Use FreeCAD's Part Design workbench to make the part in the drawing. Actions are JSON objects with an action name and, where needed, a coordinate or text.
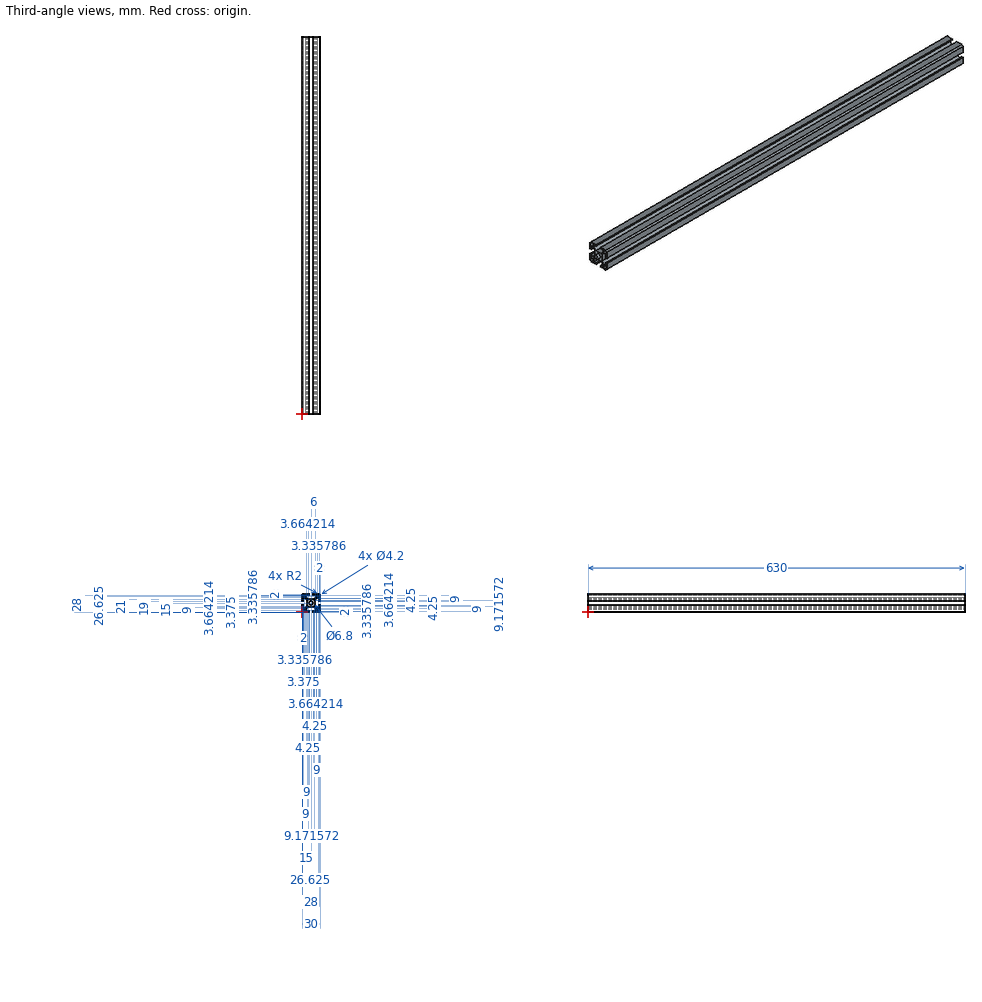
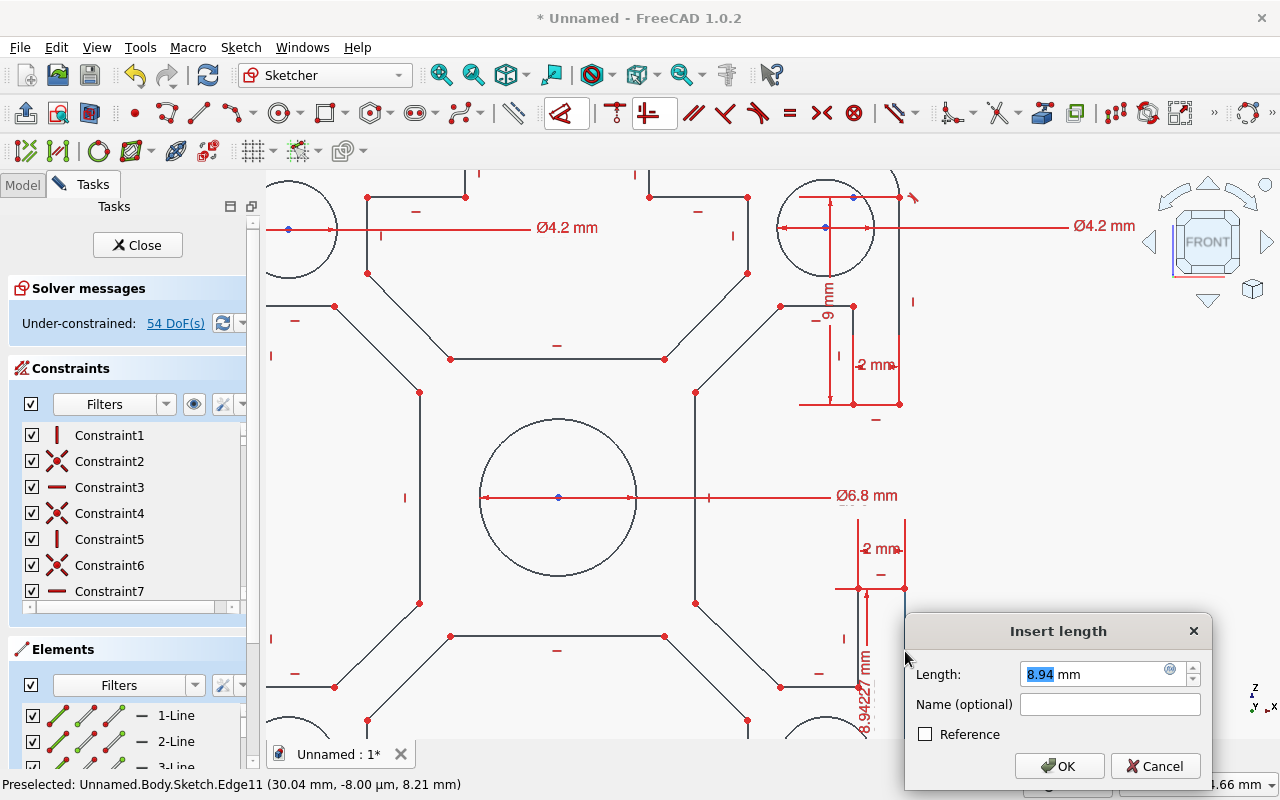
{"action": "type", "text": "9"}
{"action": "key", "text": "Return"}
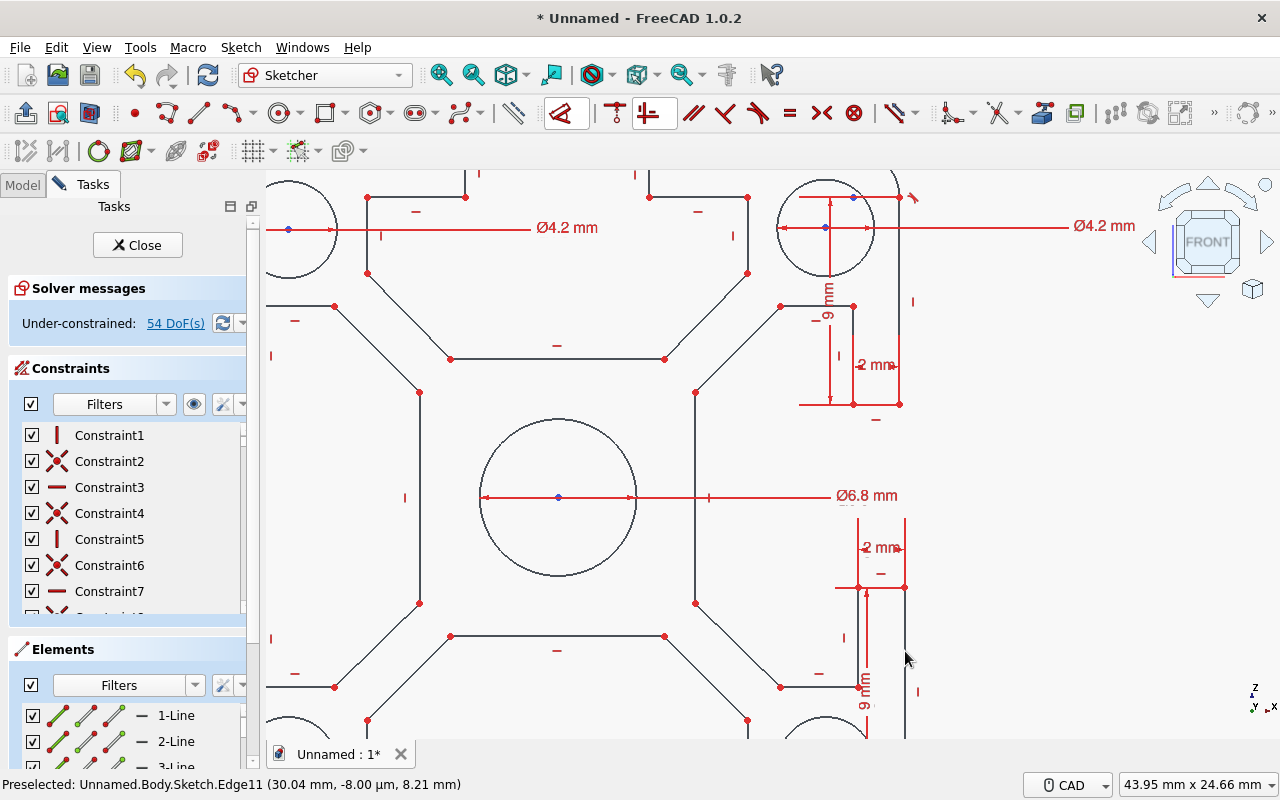
{"action": "scroll", "coordinate": [883, 405], "scroll_direction": "down", "scroll_amount": 3}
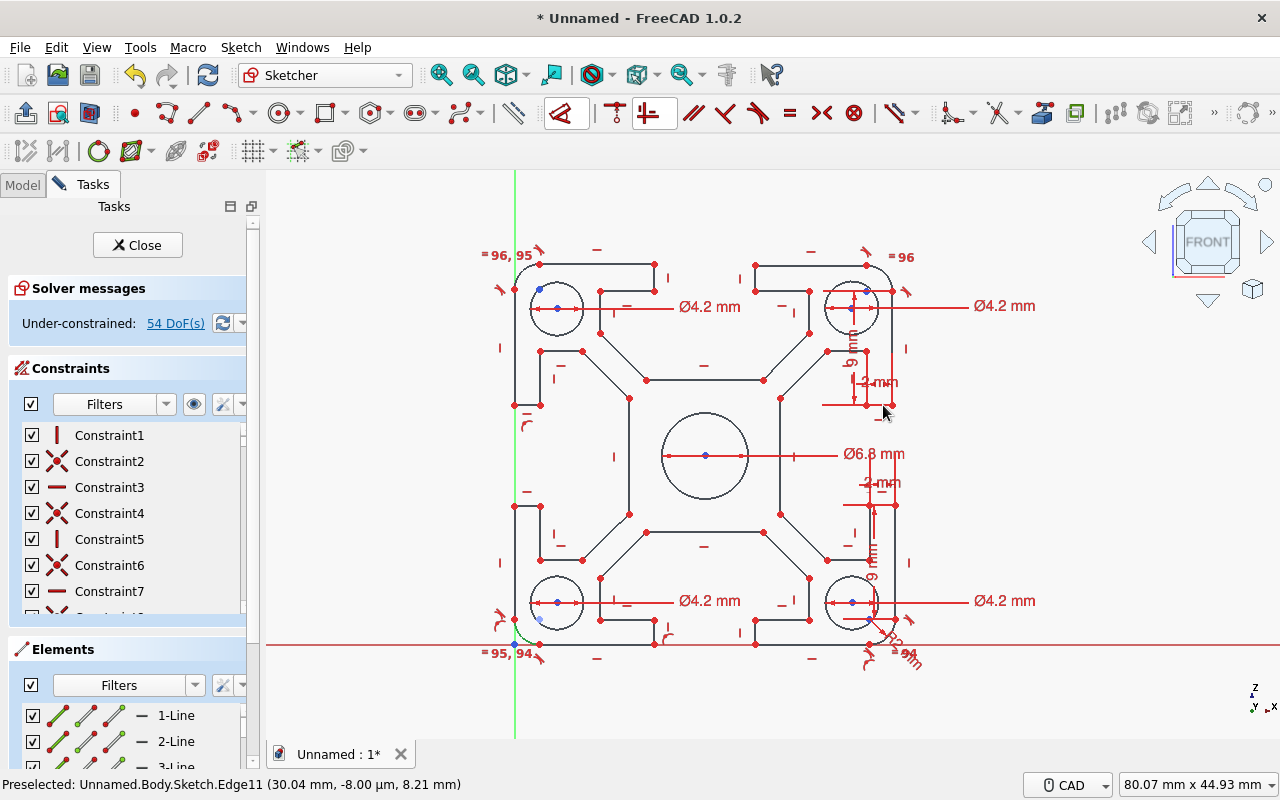
{"action": "left_click", "coordinate": [835, 645]}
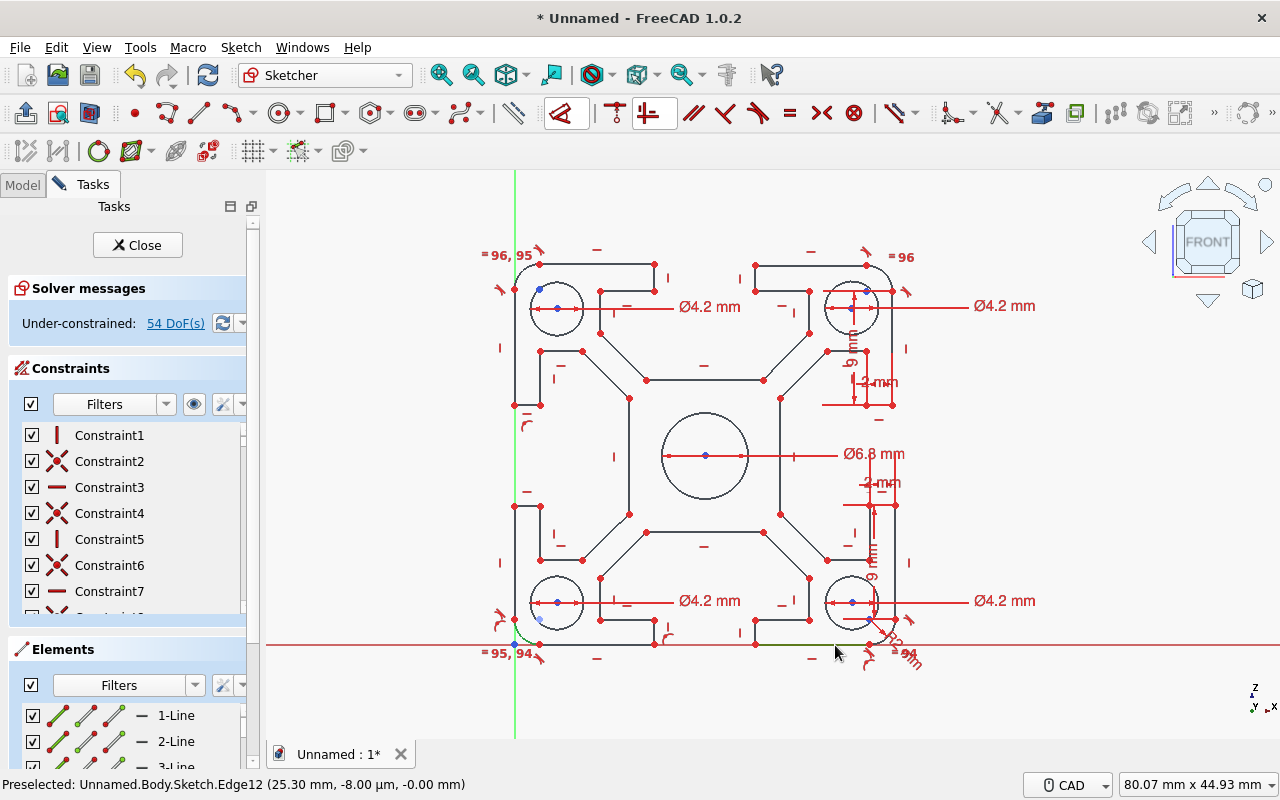
{"action": "key", "text": "l"}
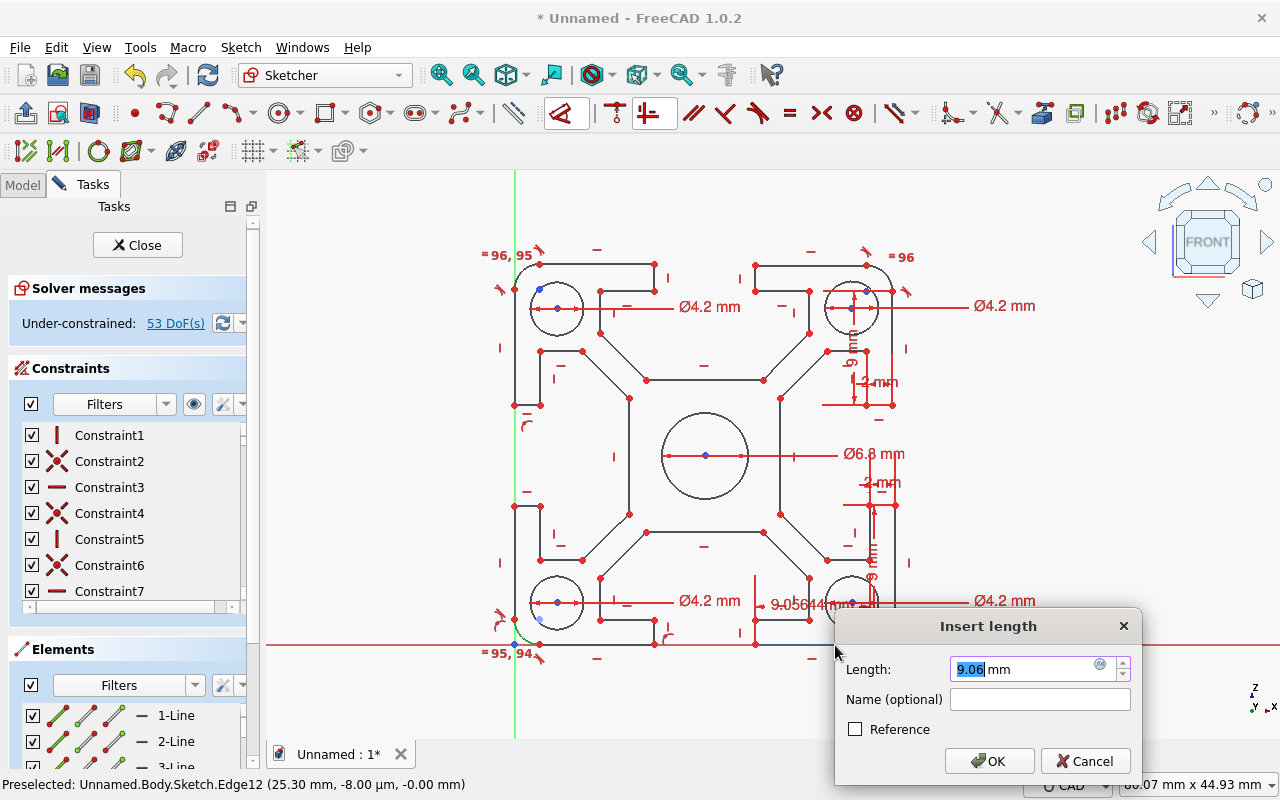
{"action": "type", "text": "9"}
{"action": "key", "text": "Return"}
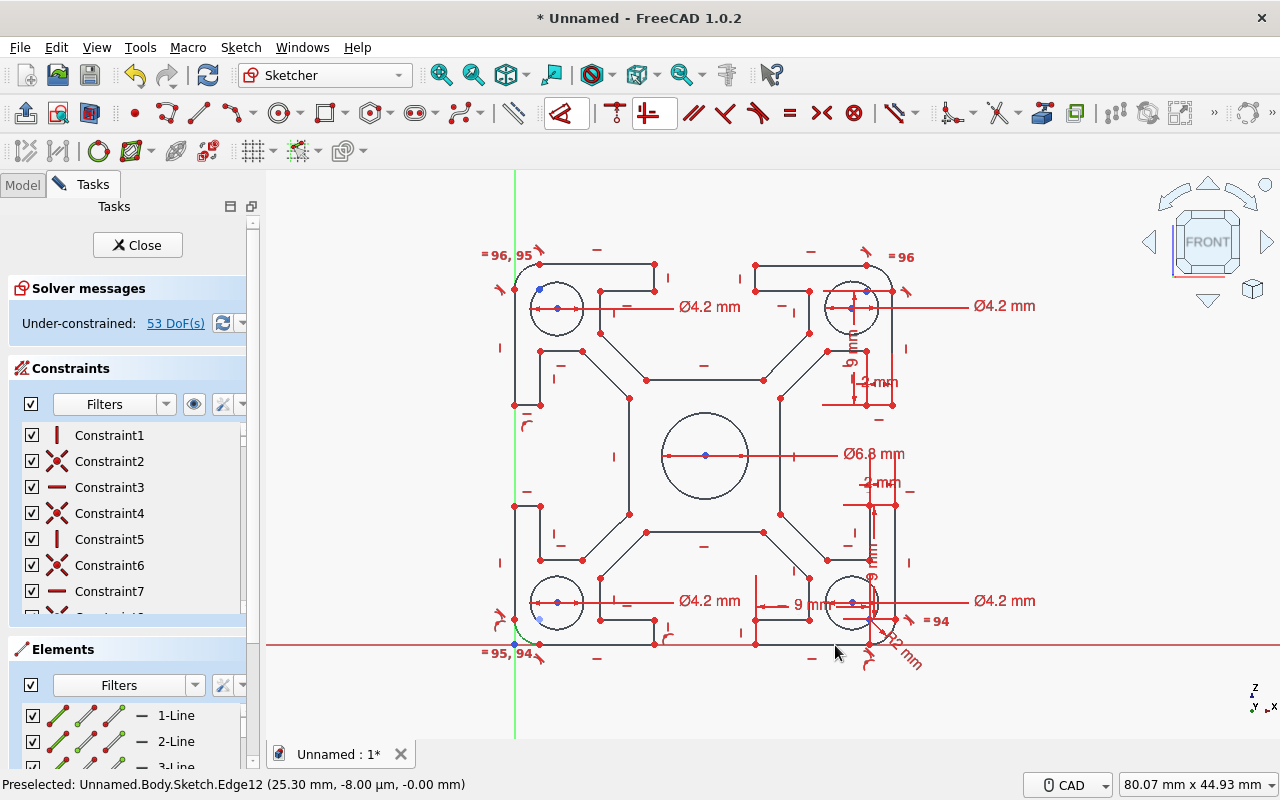
{"action": "scroll", "coordinate": [756, 635], "scroll_direction": "up", "scroll_amount": 3}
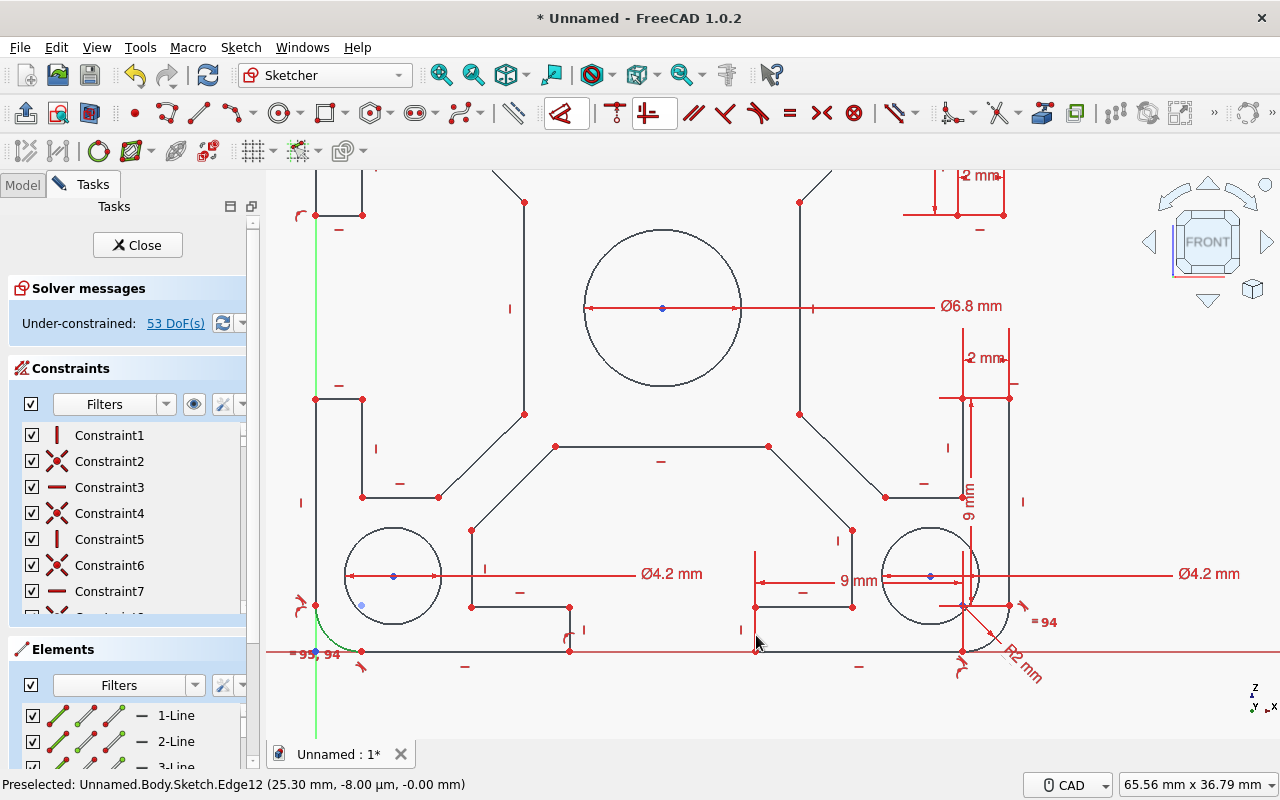
{"action": "left_click", "coordinate": [755, 634]}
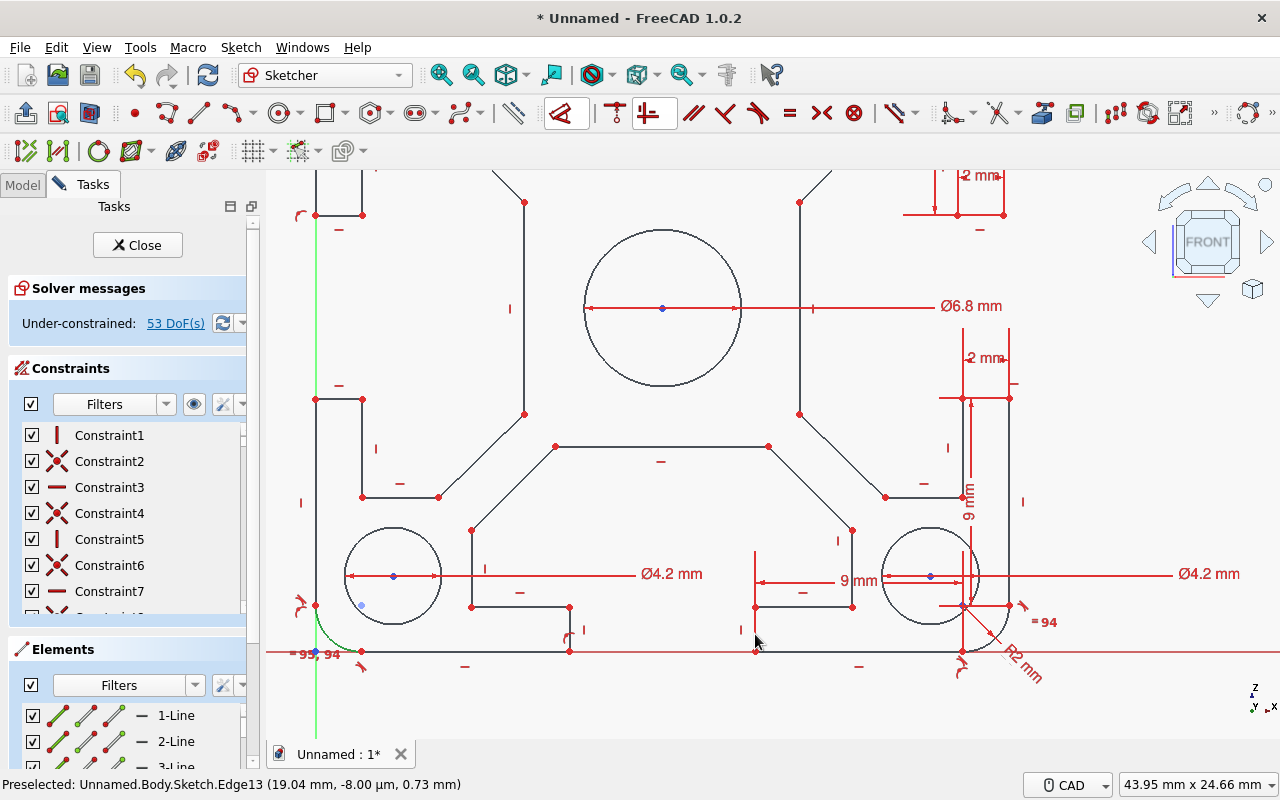
{"action": "key", "text": "i"}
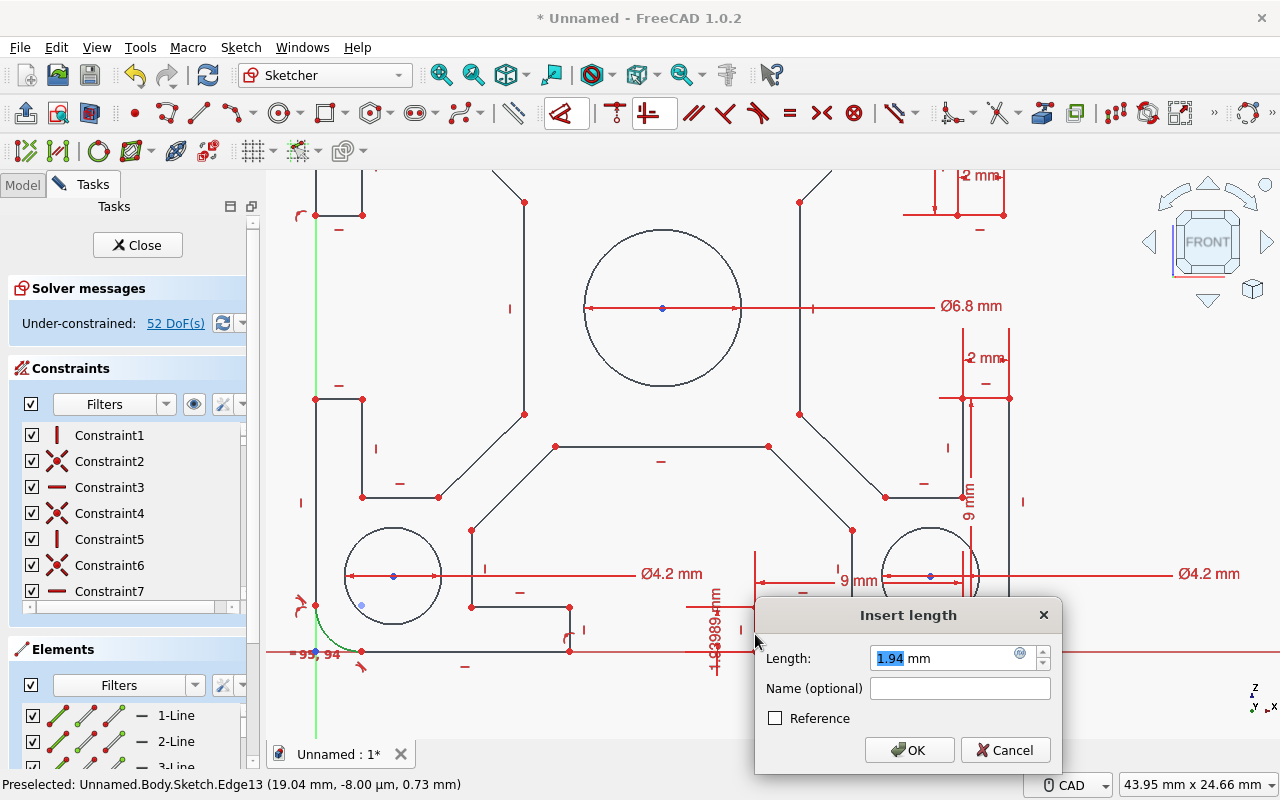
{"action": "type", "text": "2"}
{"action": "key", "text": "Return"}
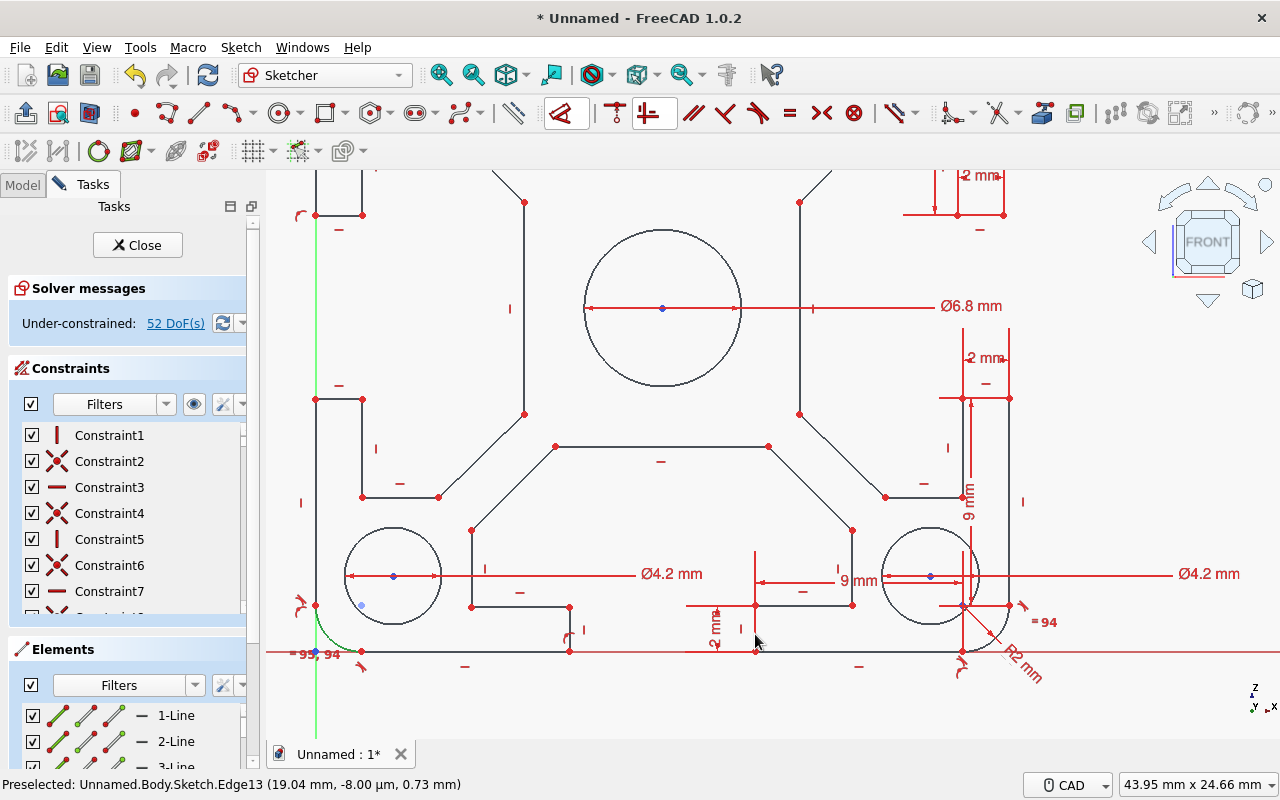
{"action": "left_click", "coordinate": [570, 621]}